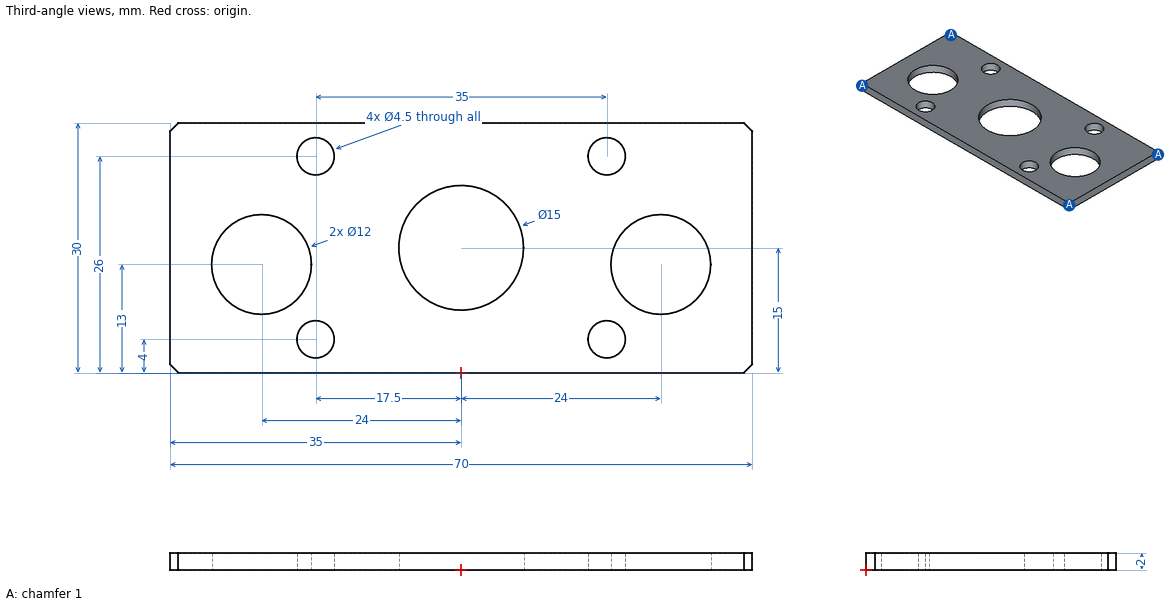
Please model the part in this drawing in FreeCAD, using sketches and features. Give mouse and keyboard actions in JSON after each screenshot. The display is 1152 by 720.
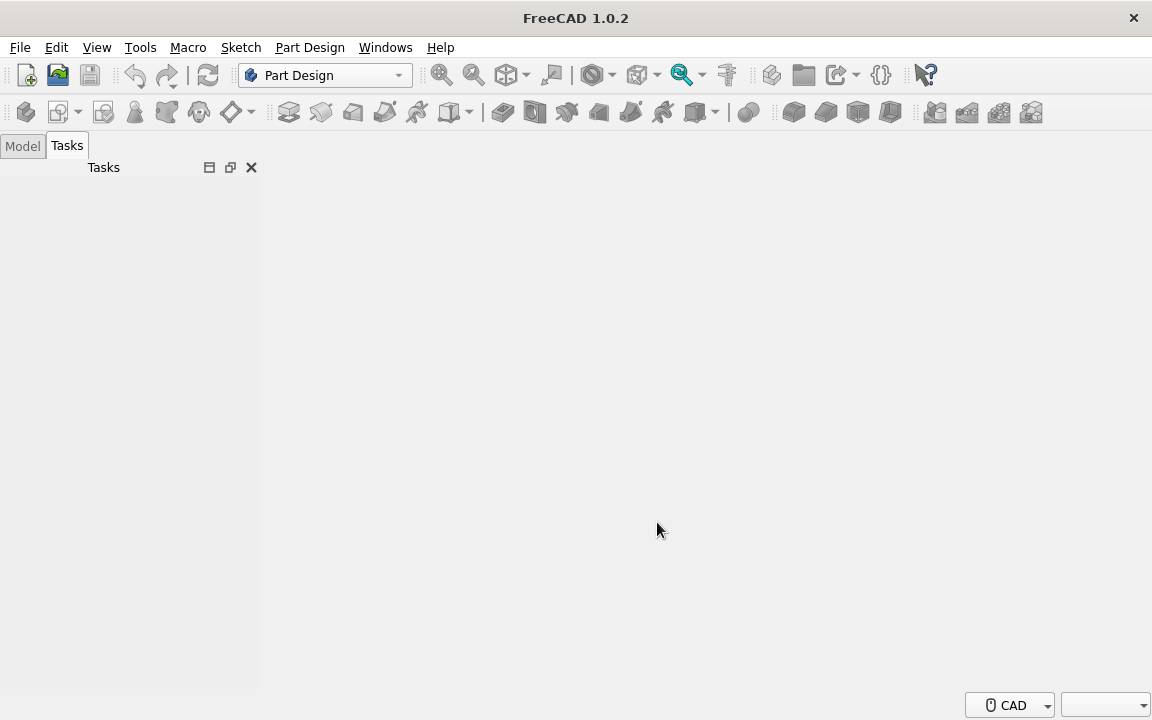
{"action": "left_click", "coordinate": [26, 76]}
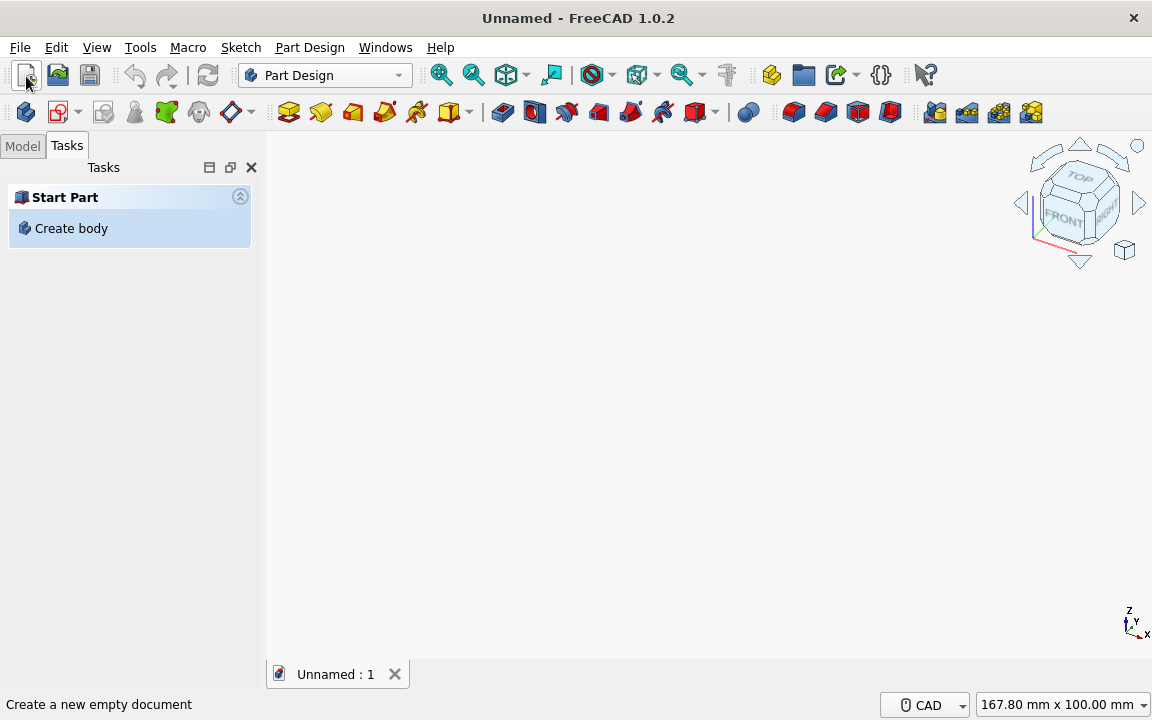
{"action": "left_click", "coordinate": [58, 112]}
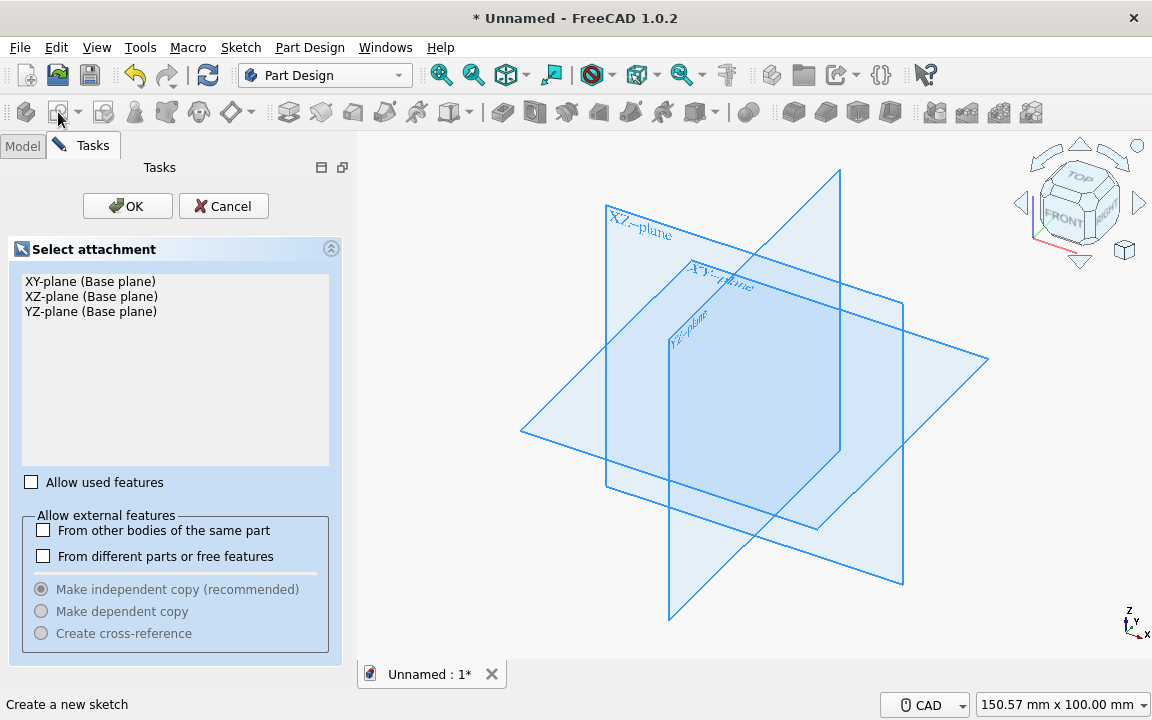
{"action": "left_click", "coordinate": [82, 282]}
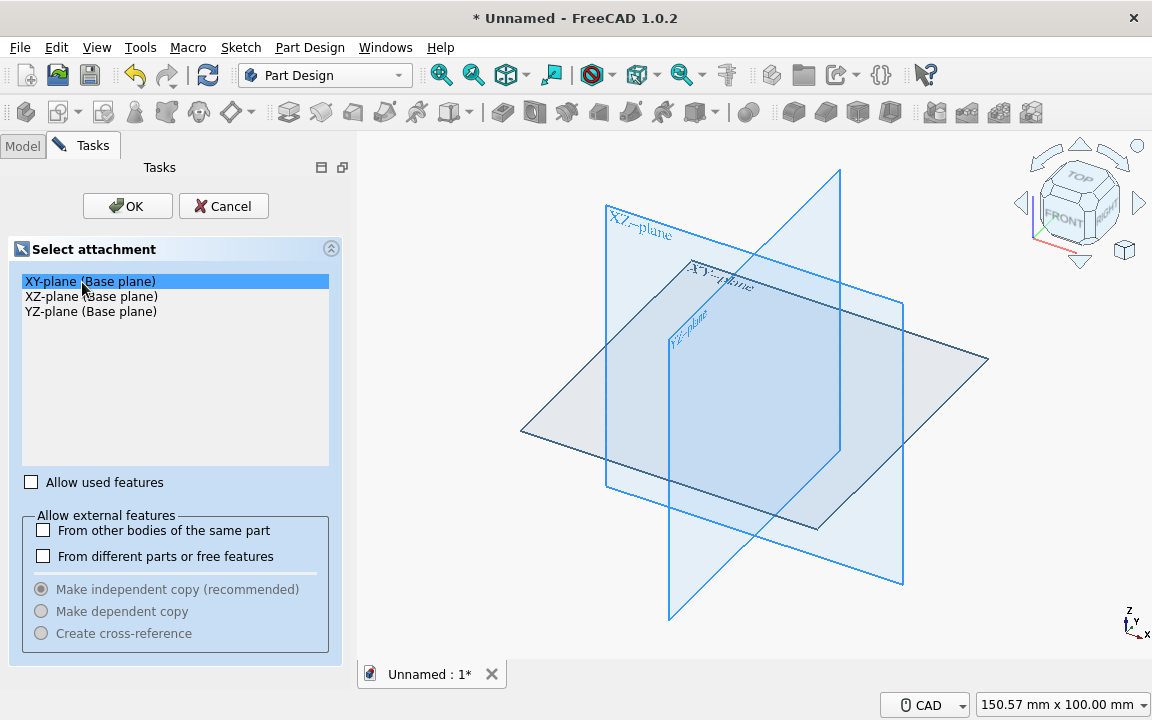
{"action": "left_click", "coordinate": [128, 206]}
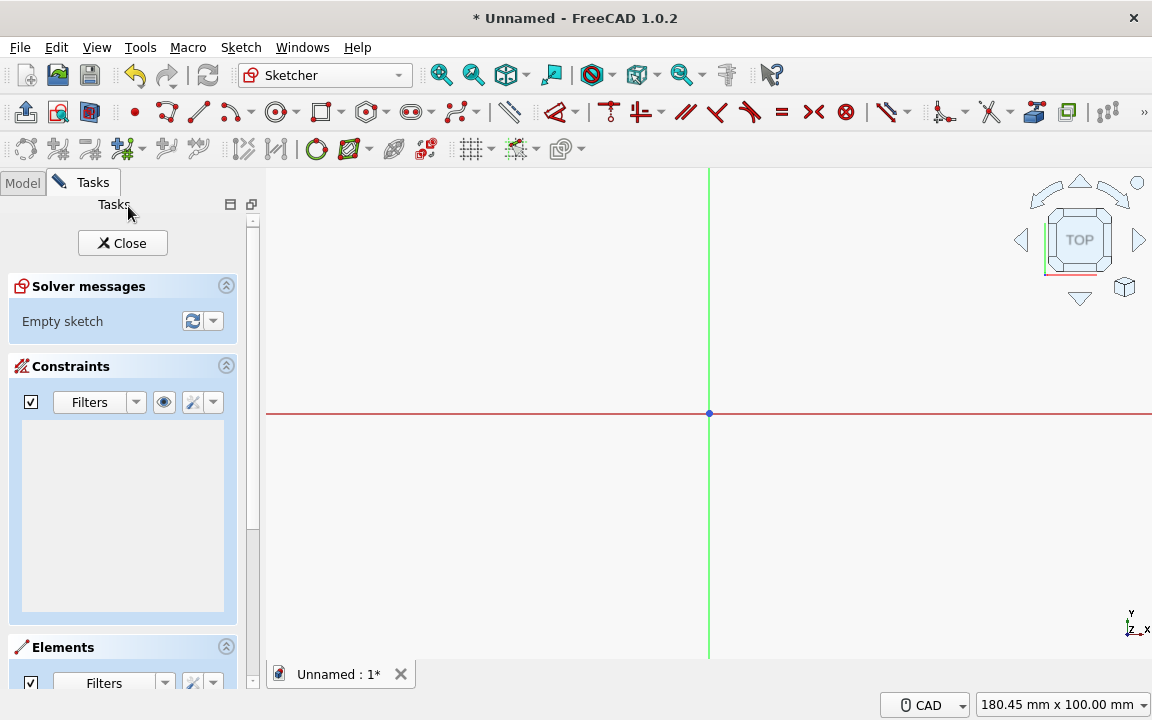
{"action": "scroll", "coordinate": [848, 196], "scroll_direction": "up", "scroll_amount": 2}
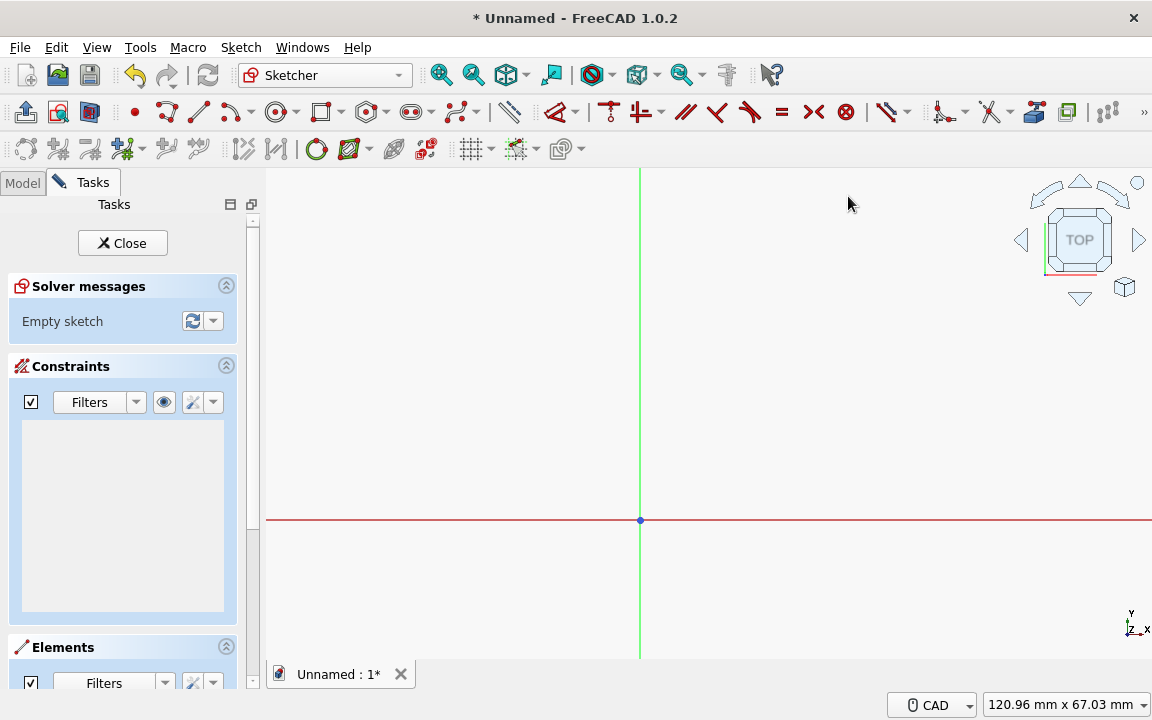
{"action": "left_click", "coordinate": [322, 112]}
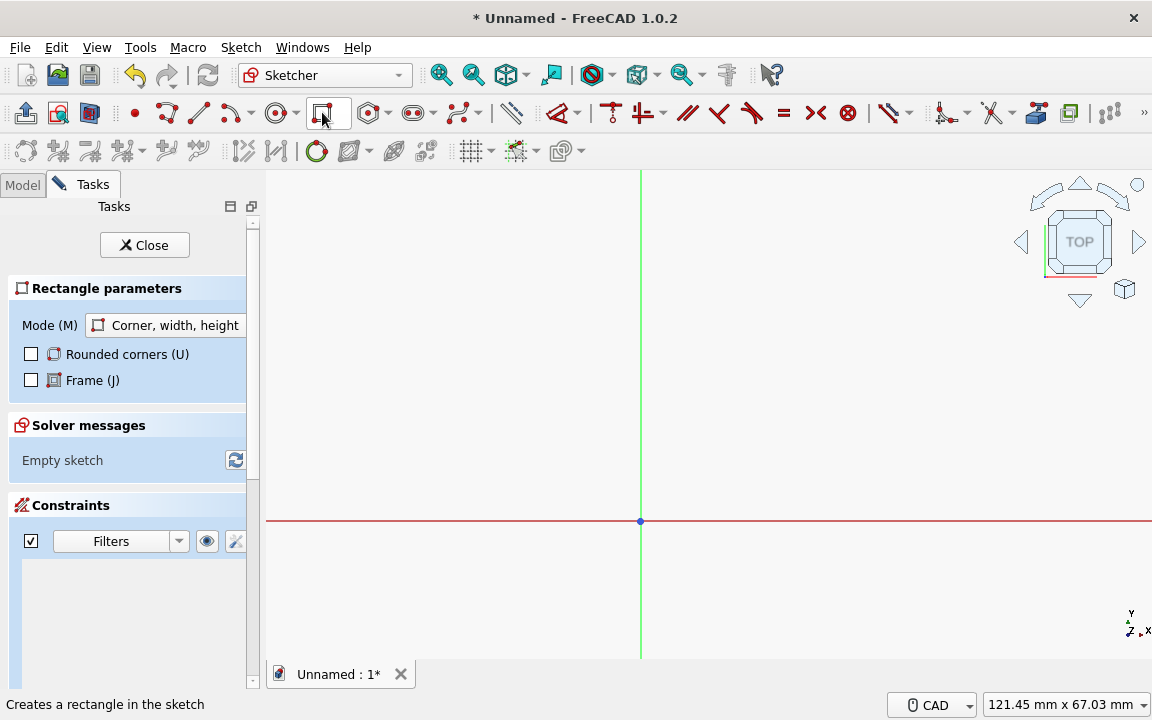
{"action": "left_click", "coordinate": [385, 302]}
{"action": "left_click", "coordinate": [896, 521]}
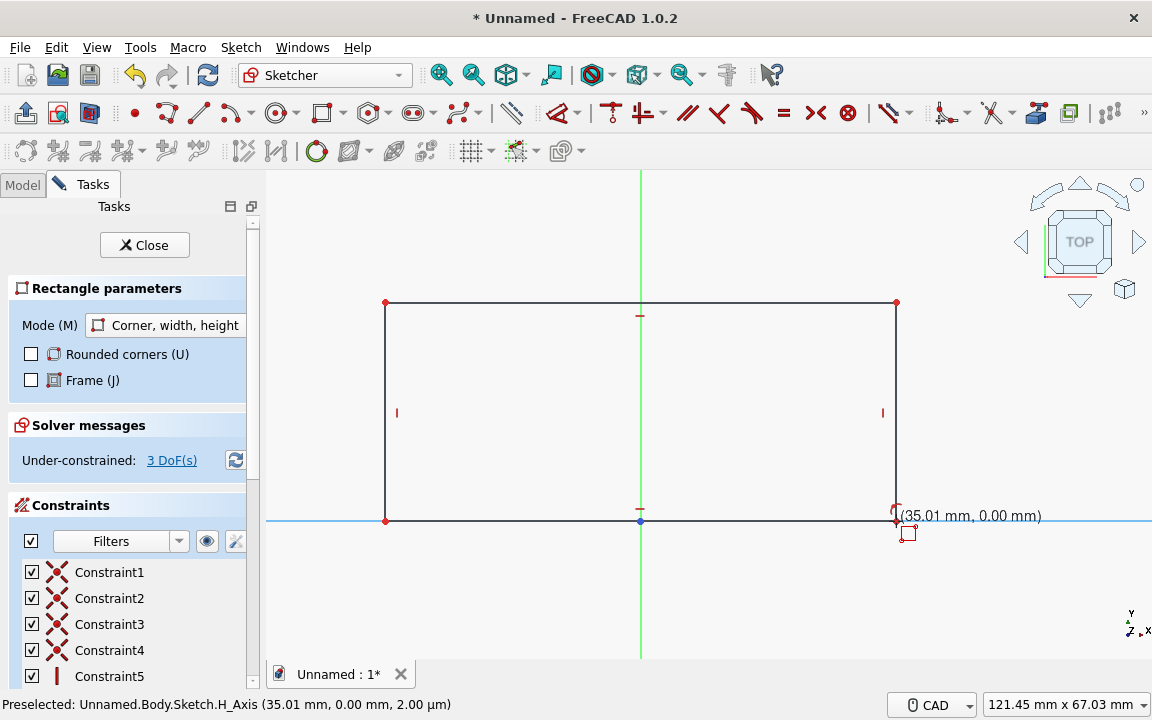
{"action": "left_click", "coordinate": [276, 114]}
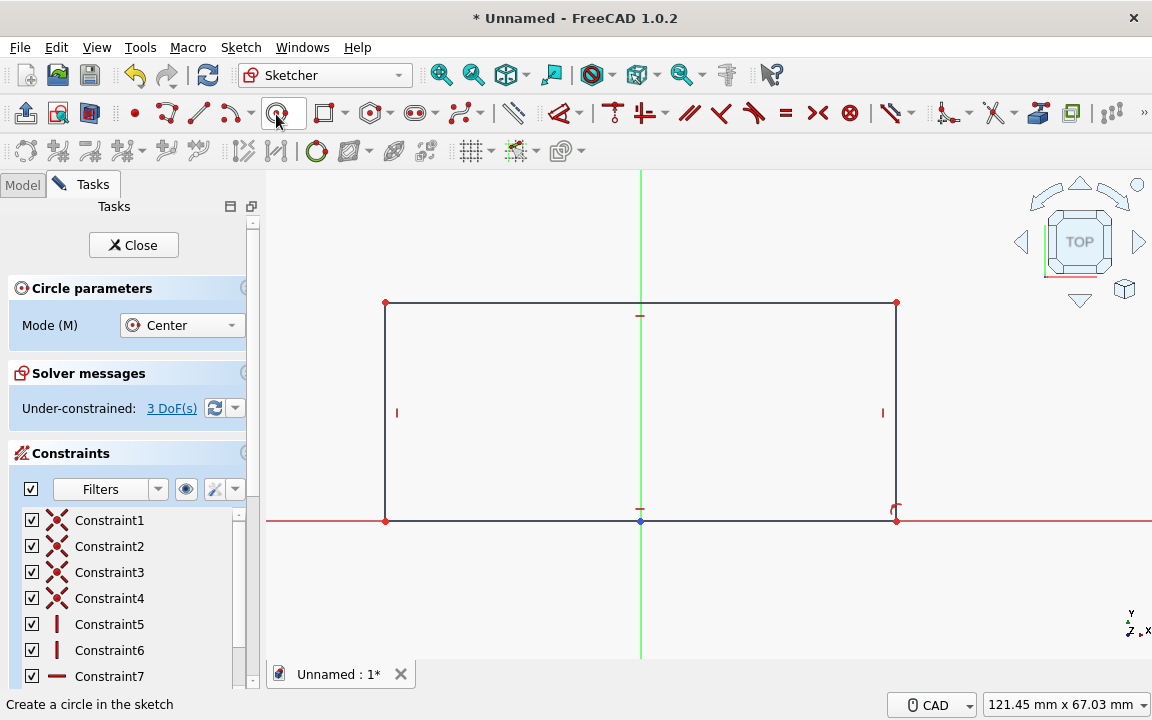
{"action": "left_click", "coordinate": [466, 426]}
{"action": "left_click", "coordinate": [496, 395]}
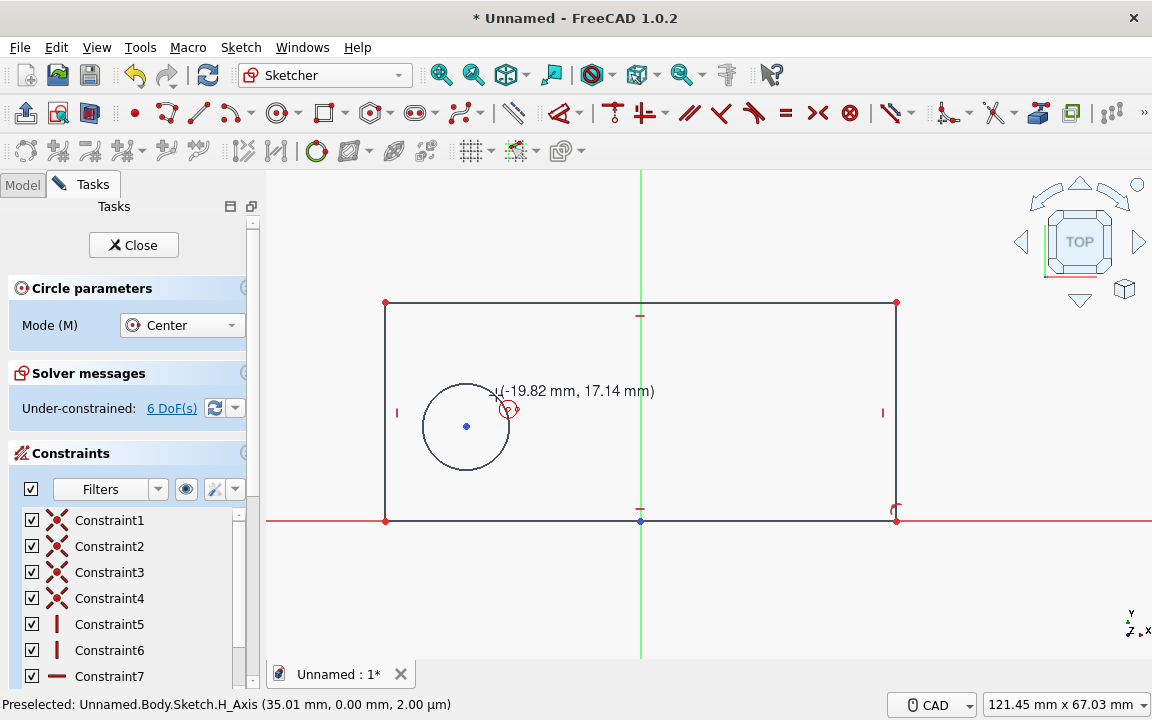
{"action": "left_click", "coordinate": [816, 426]}
{"action": "left_click", "coordinate": [847, 395]}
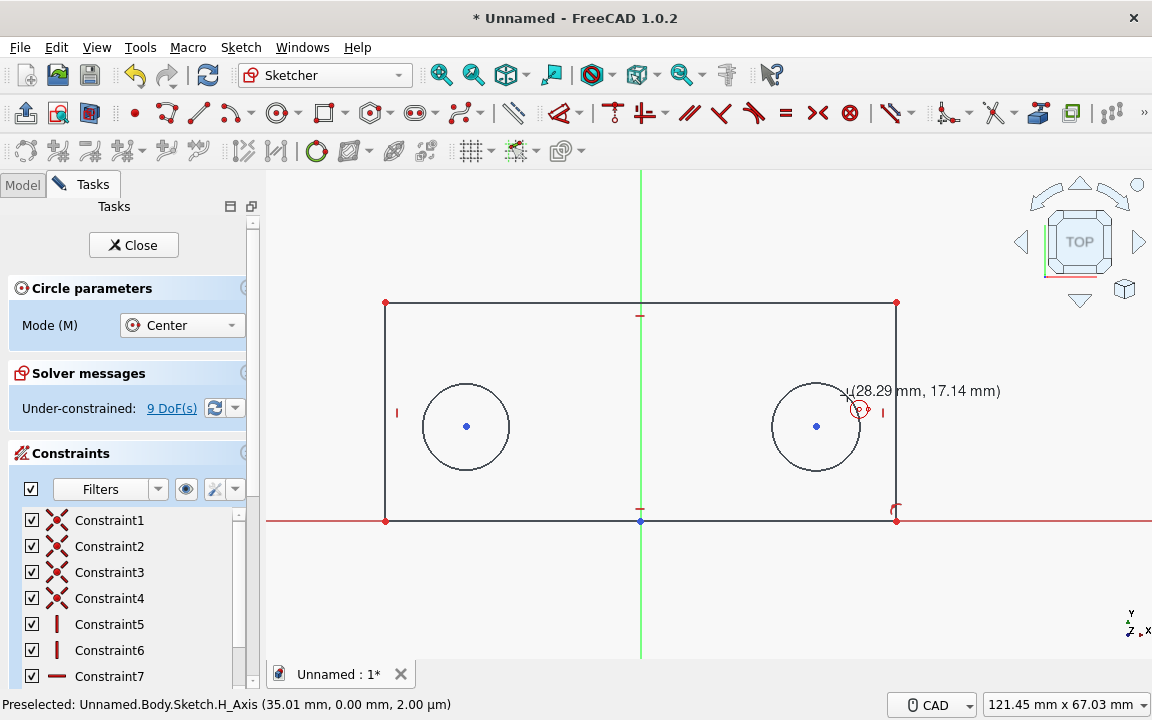
{"action": "left_click", "coordinate": [641, 412]}
{"action": "left_click", "coordinate": [679, 373]}
{"action": "key", "text": "Escape"}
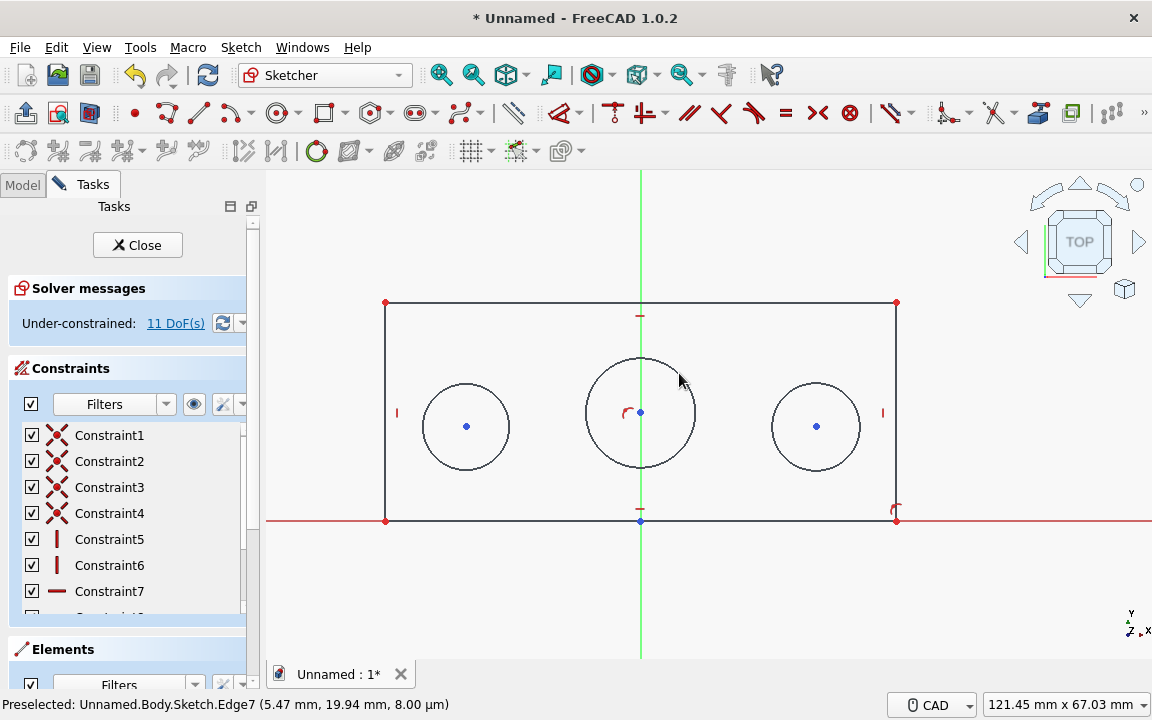
{"action": "left_click", "coordinate": [496, 396]}